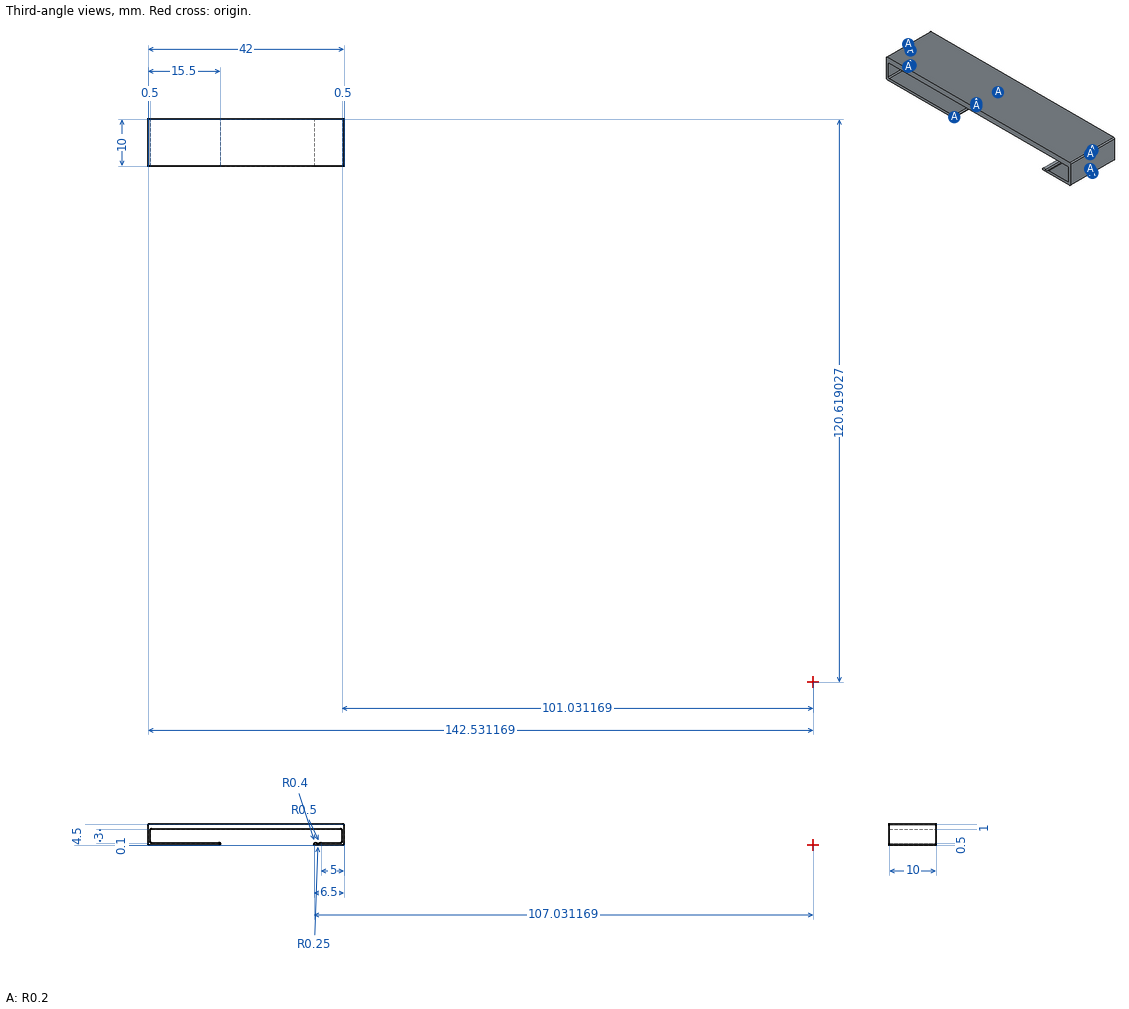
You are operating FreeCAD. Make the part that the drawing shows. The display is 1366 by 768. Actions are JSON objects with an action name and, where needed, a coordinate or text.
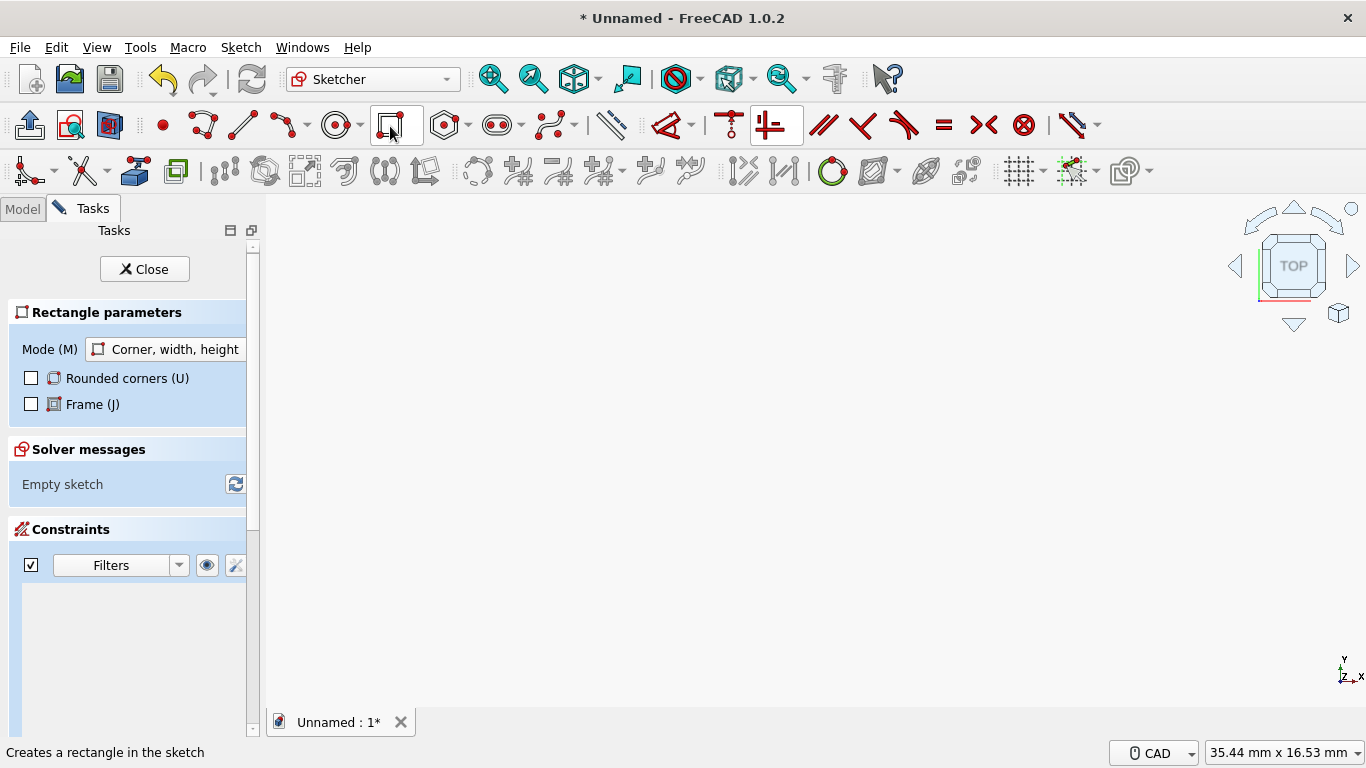
{"action": "left_click", "coordinate": [507, 294]}
{"action": "left_click", "coordinate": [988, 605]}
{"action": "key", "text": "Escape"}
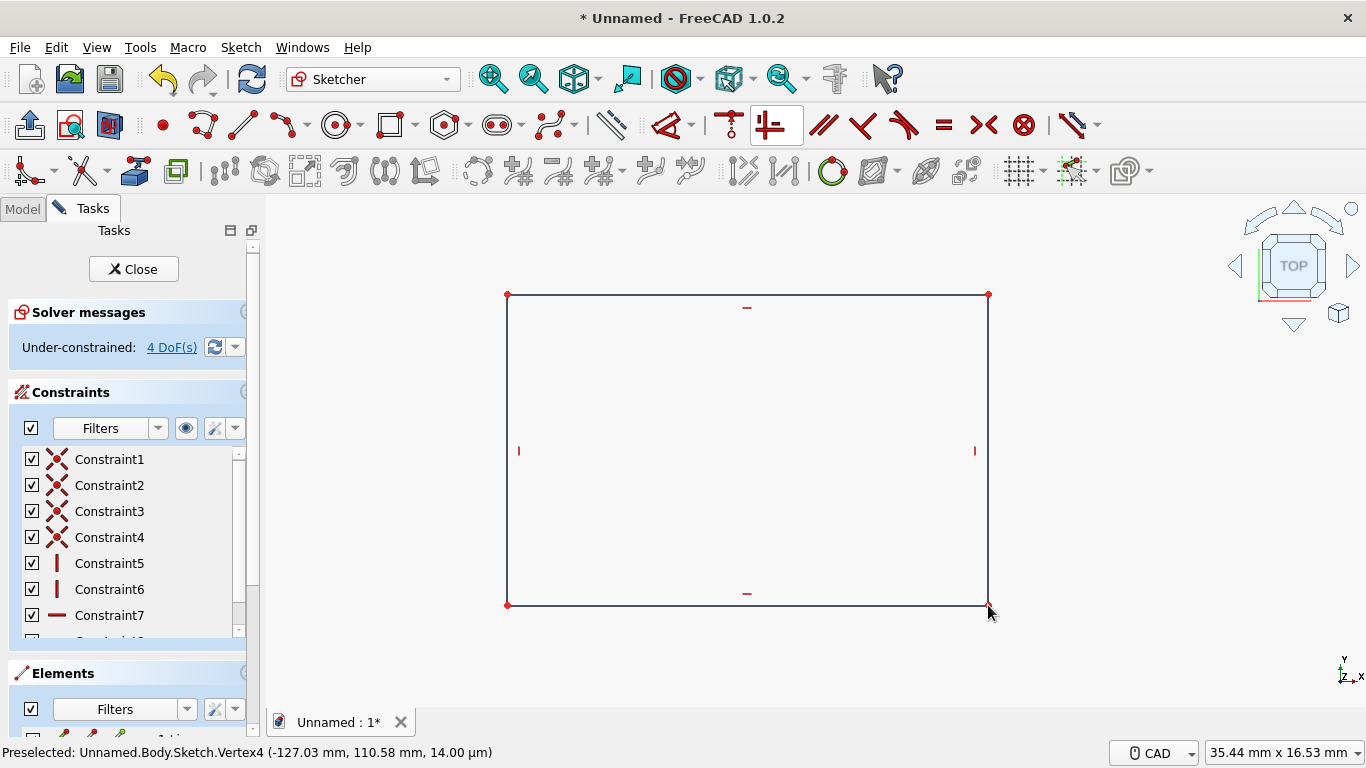
{"action": "left_click", "coordinate": [666, 126]}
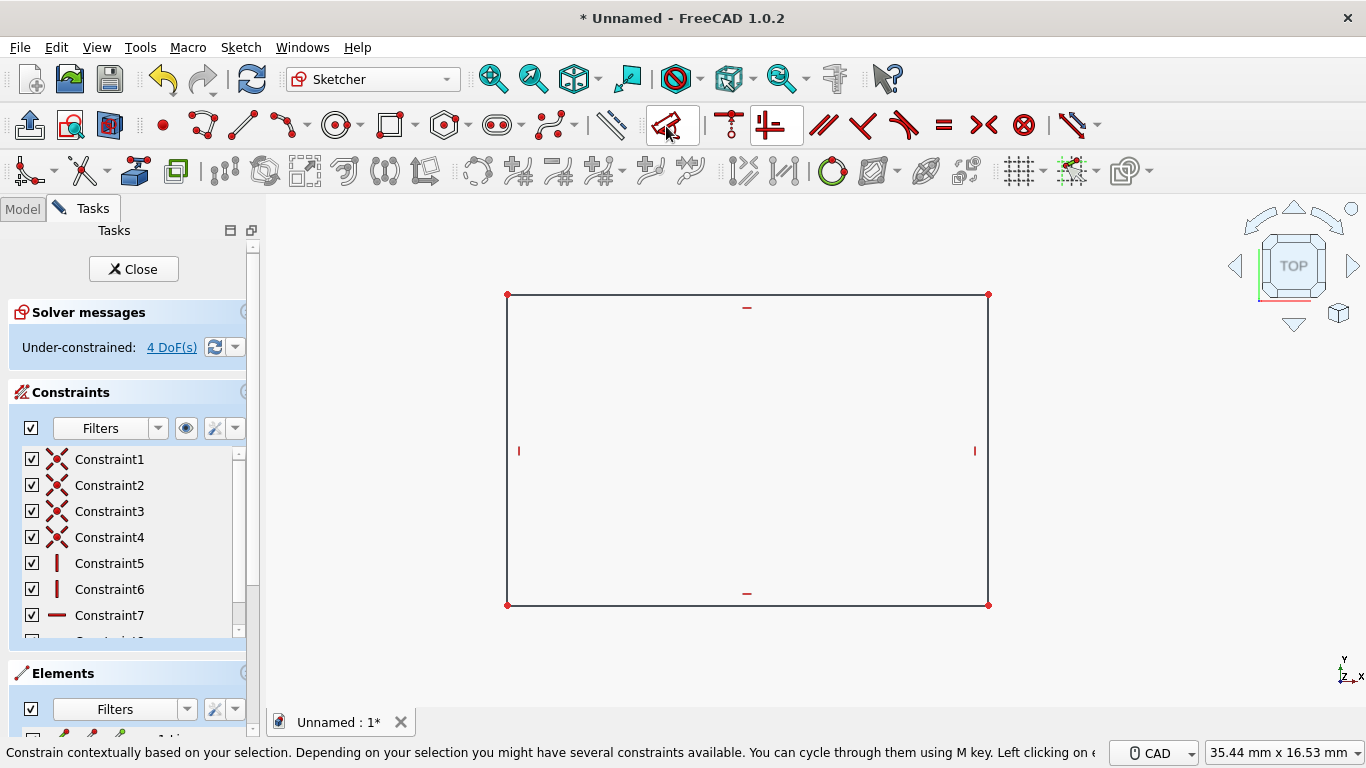
{"action": "left_click", "coordinate": [507, 388]}
{"action": "left_click", "coordinate": [473, 450]}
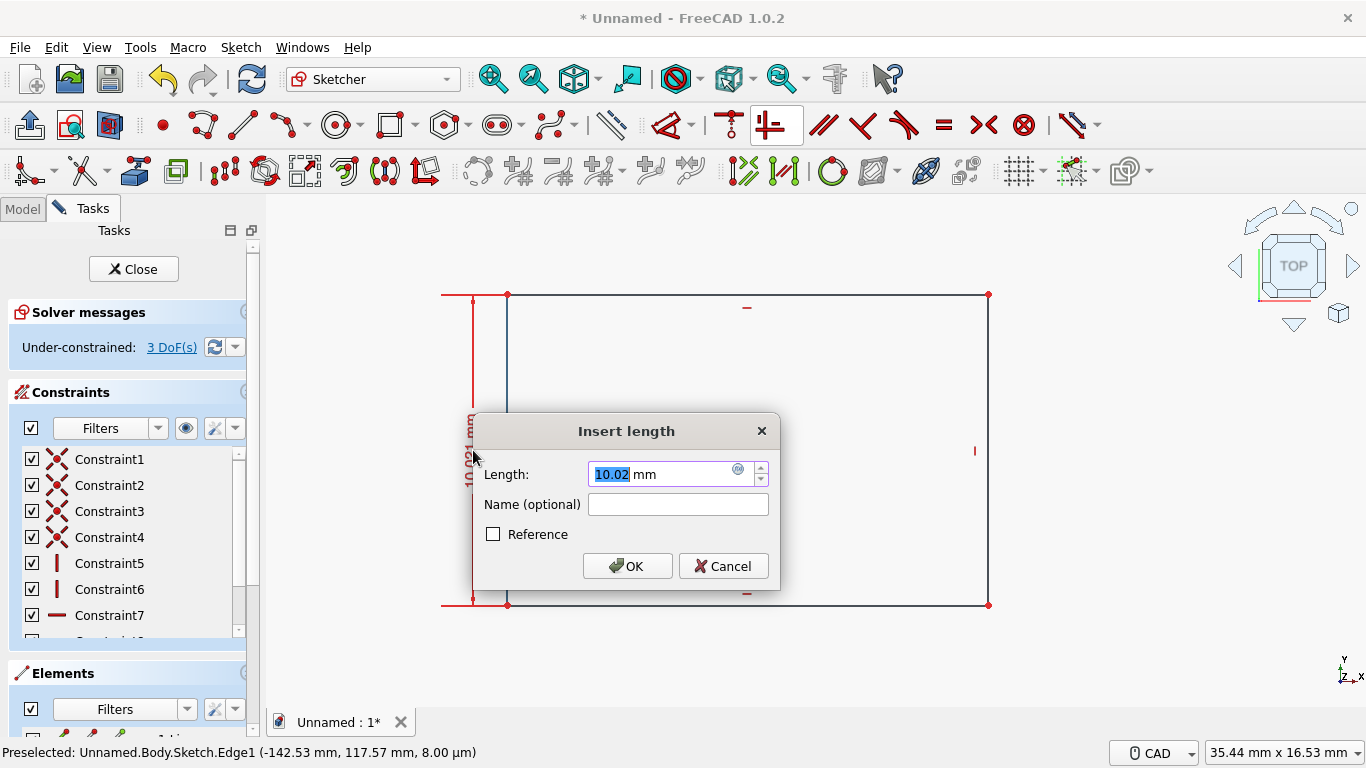
{"action": "type", "text": "10"}
{"action": "key", "text": "Return"}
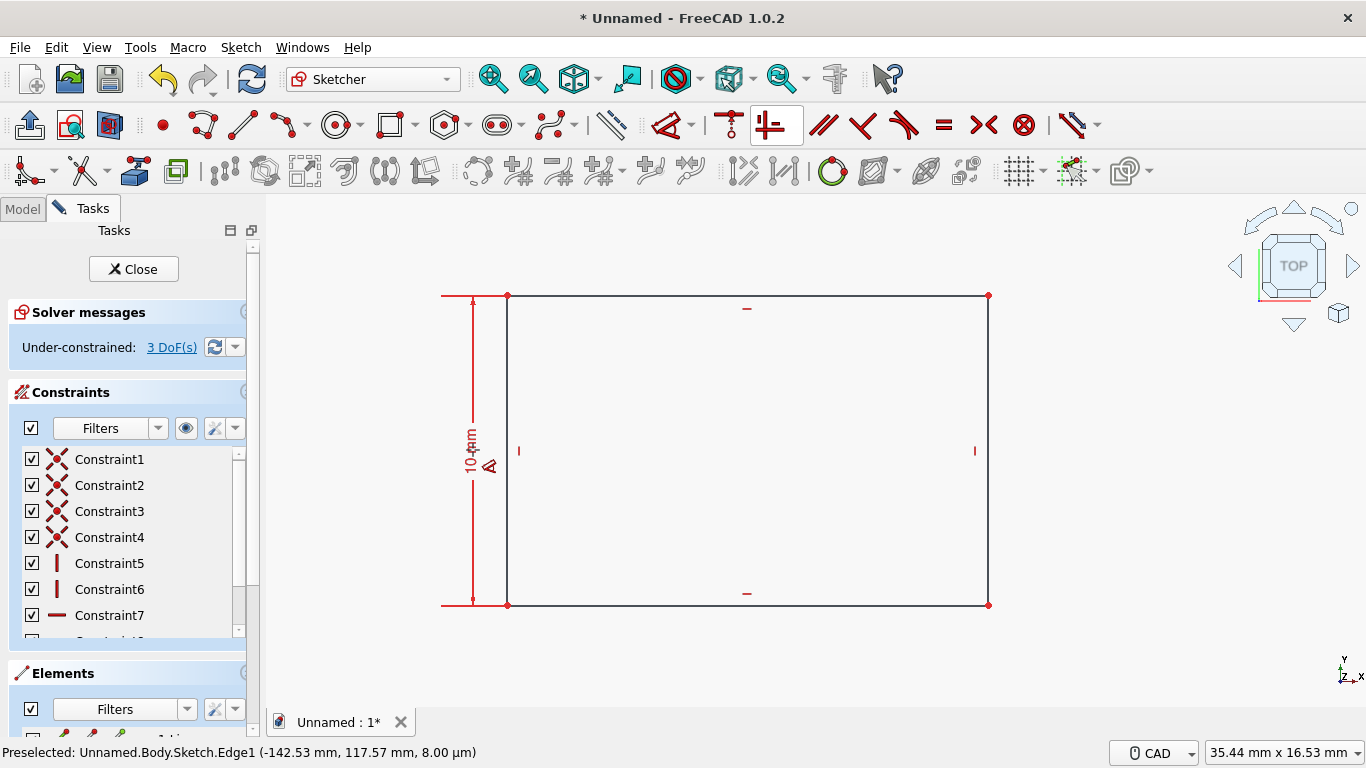
{"action": "left_click", "coordinate": [651, 606]}
{"action": "left_click", "coordinate": [747, 640]}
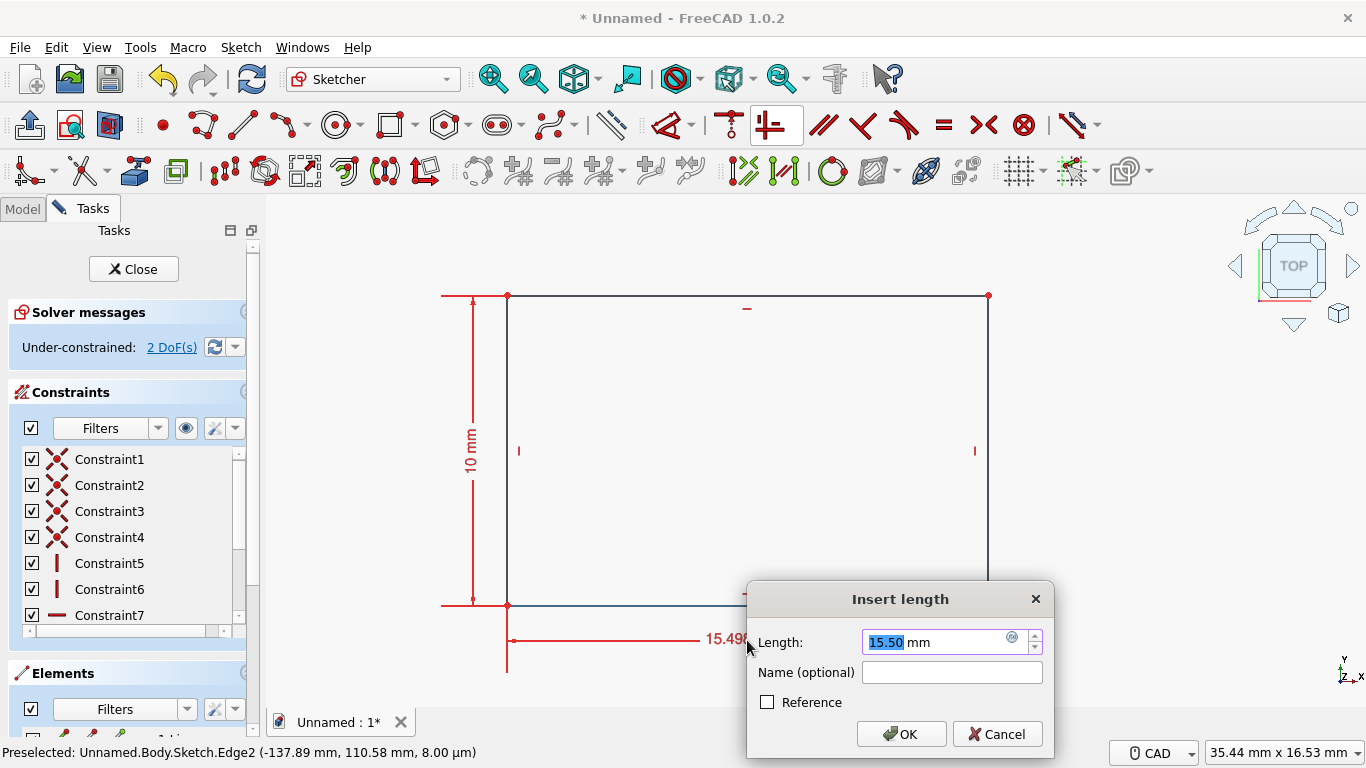
{"action": "type", "text": "15.5"}
{"action": "key", "text": "Return"}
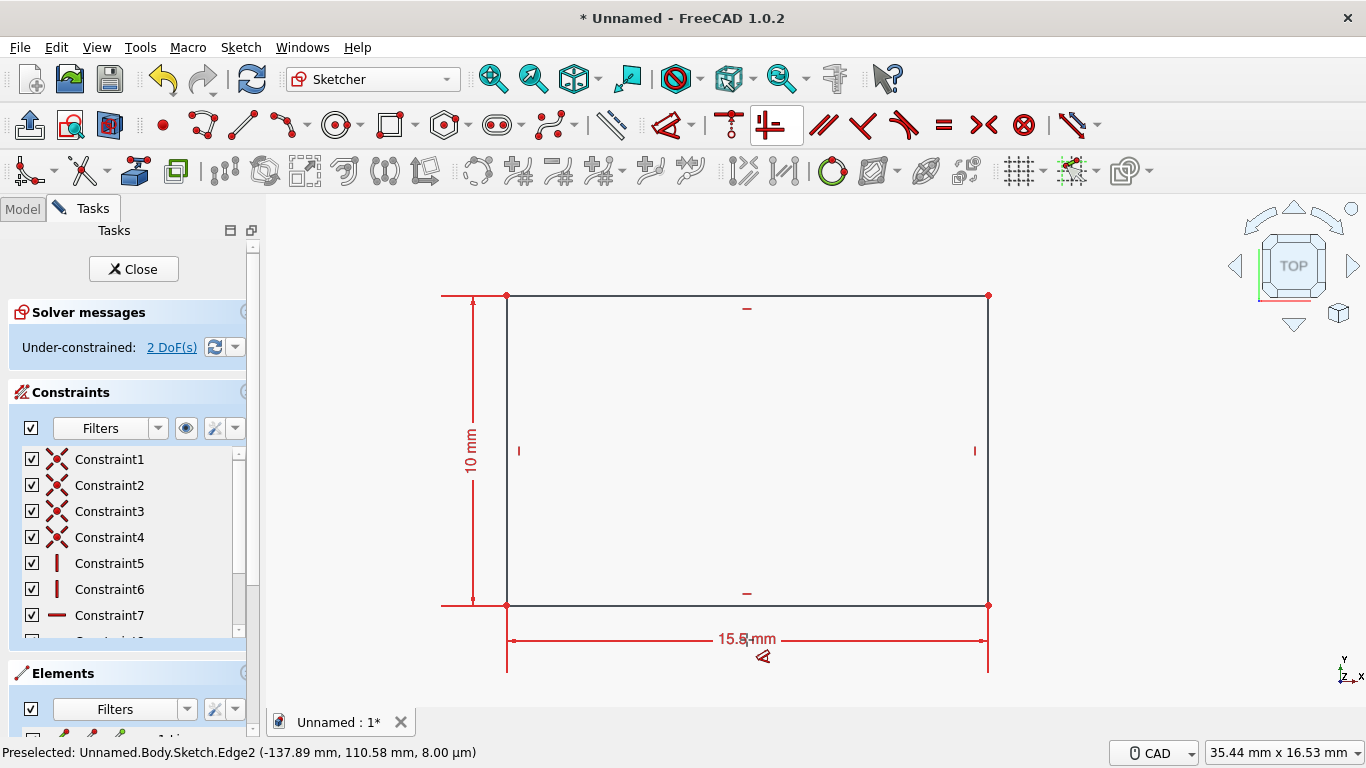
{"action": "left_click", "coordinate": [507, 296]}
{"action": "left_click", "coordinate": [854, 262]}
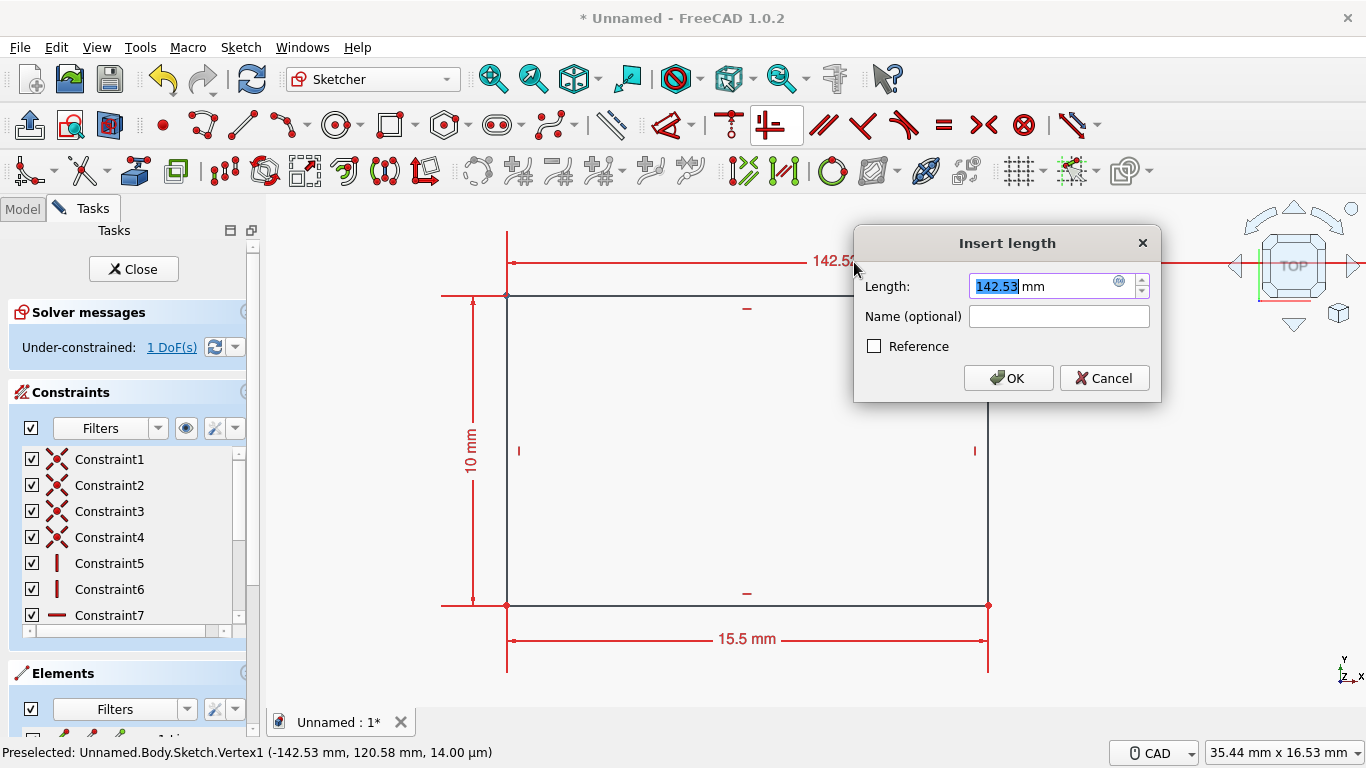
{"action": "type", "text": "142.531169"}
{"action": "key", "text": "Return"}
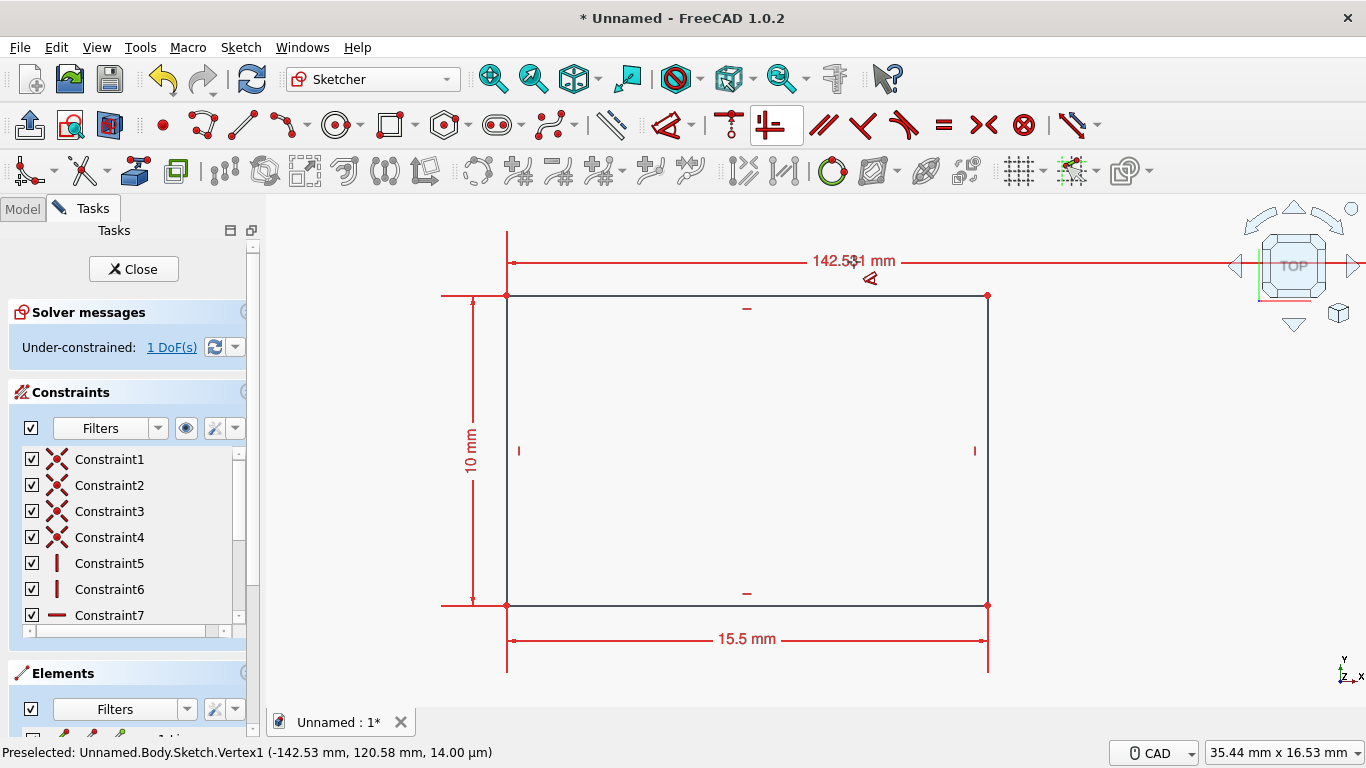
{"action": "left_click", "coordinate": [507, 296]}
{"action": "left_click", "coordinate": [473, 487]}